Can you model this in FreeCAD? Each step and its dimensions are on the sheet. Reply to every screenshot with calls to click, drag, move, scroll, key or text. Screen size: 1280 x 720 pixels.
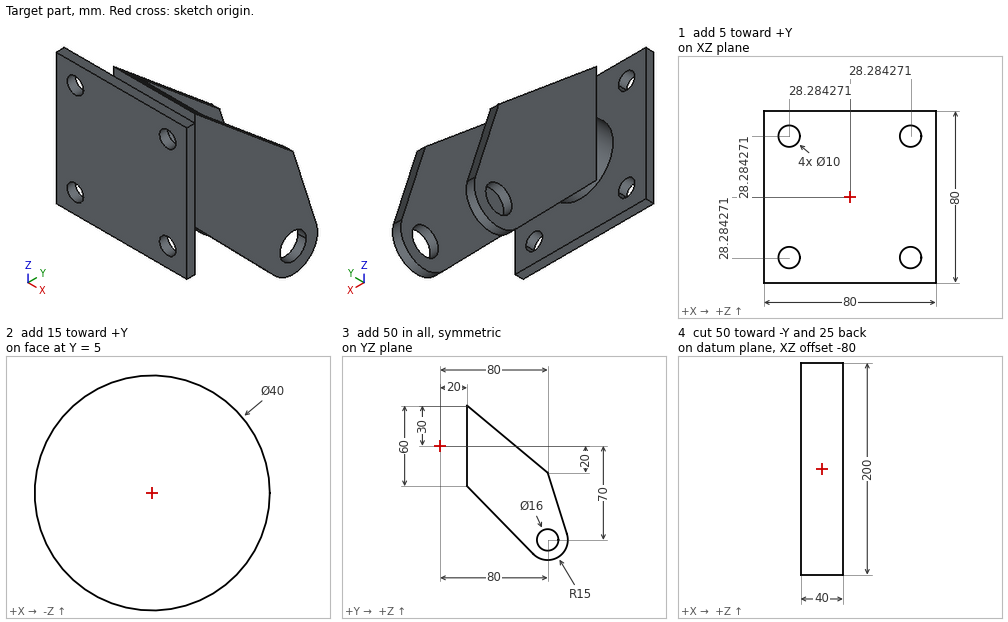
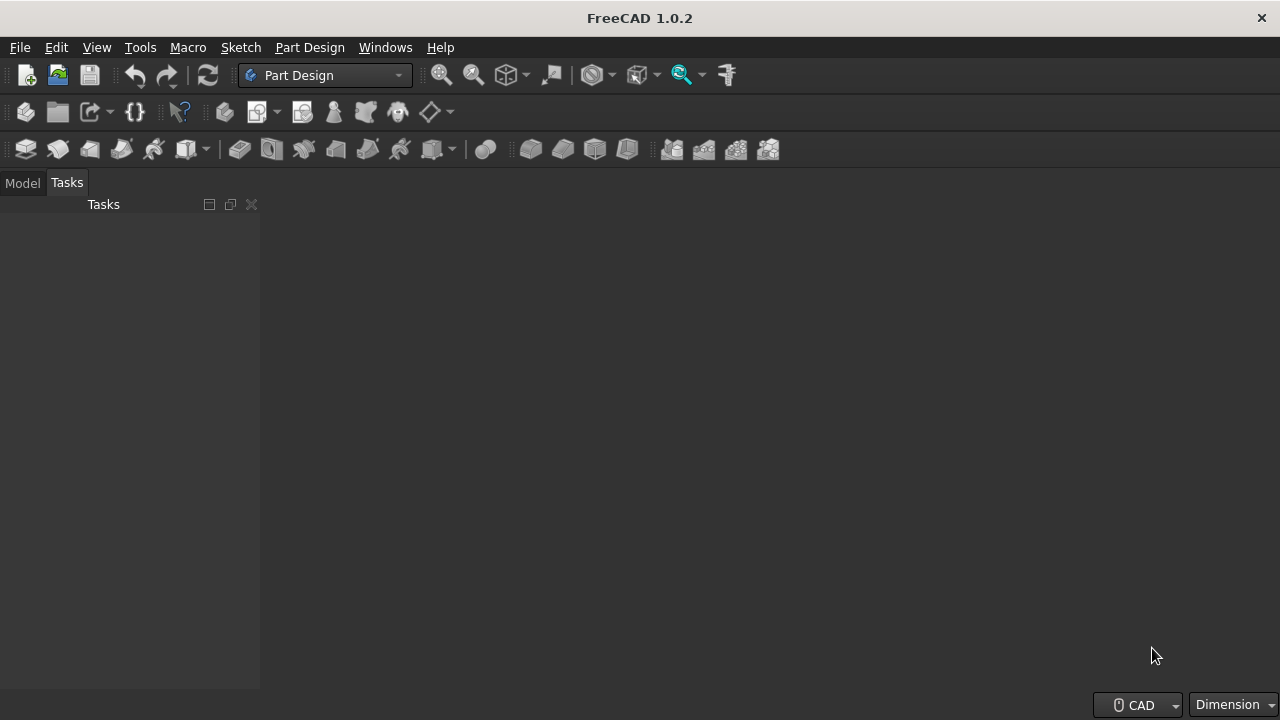
click(26, 76)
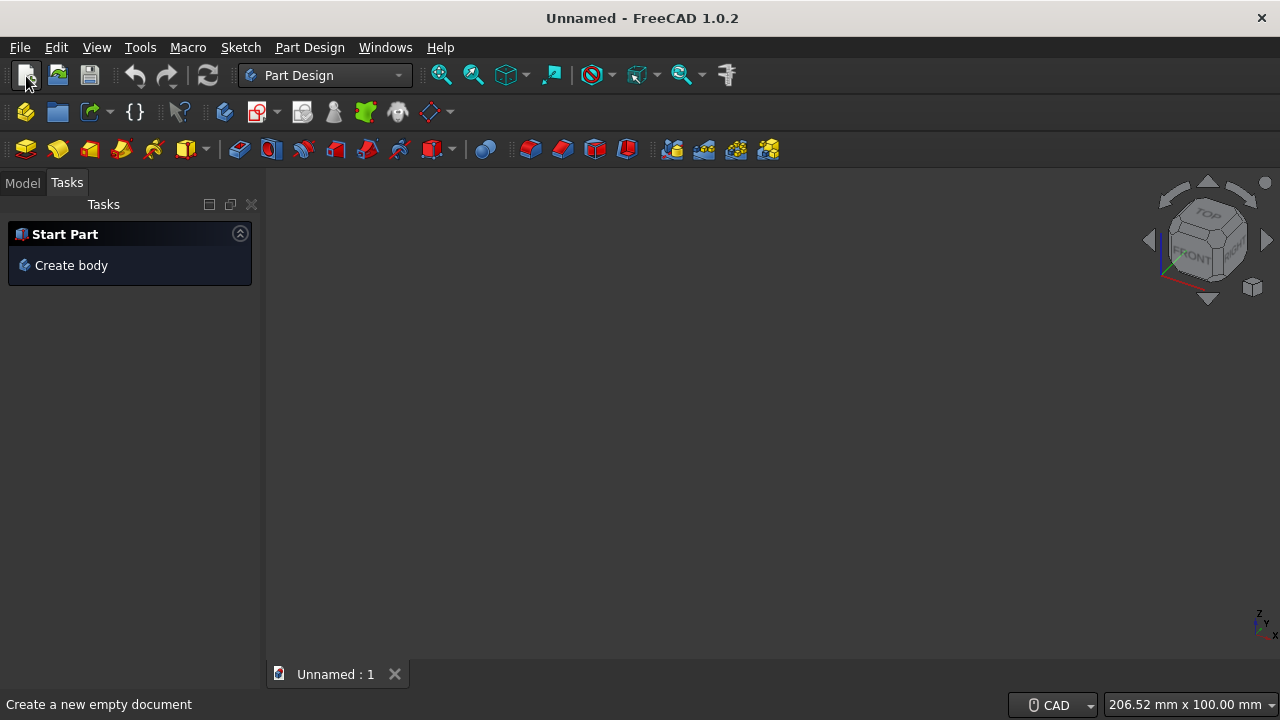
click(258, 112)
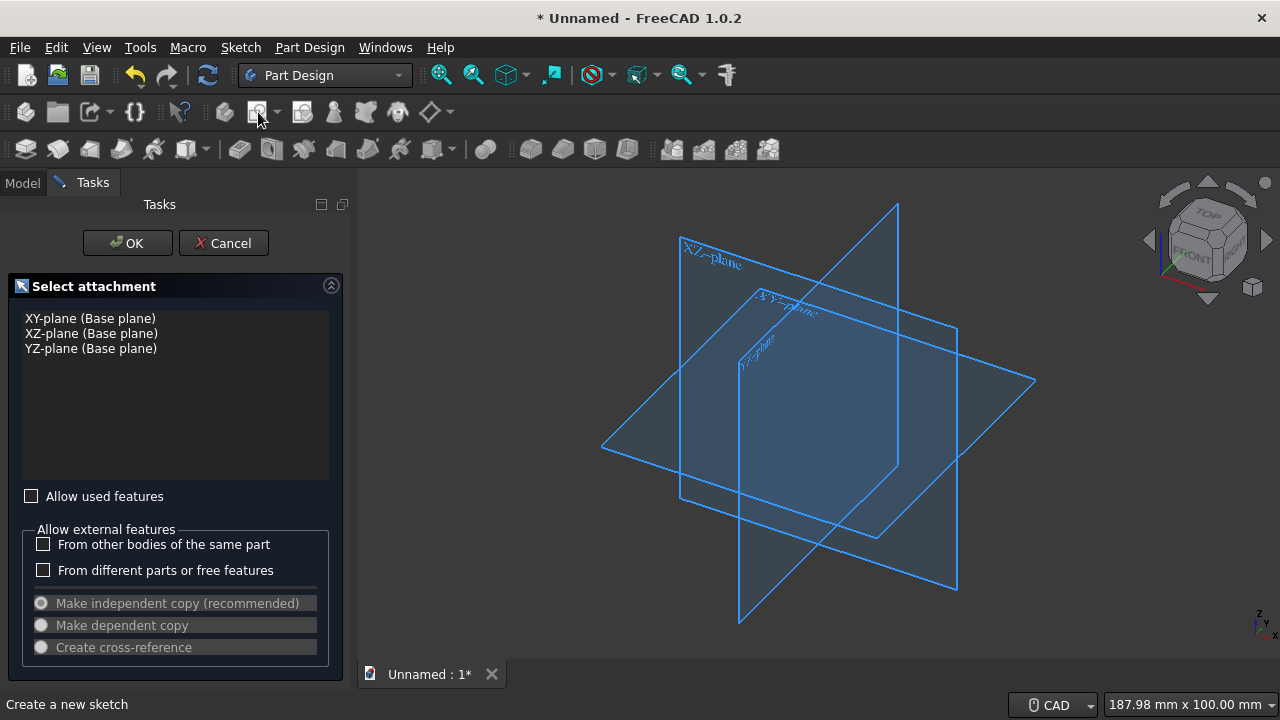
click(82, 334)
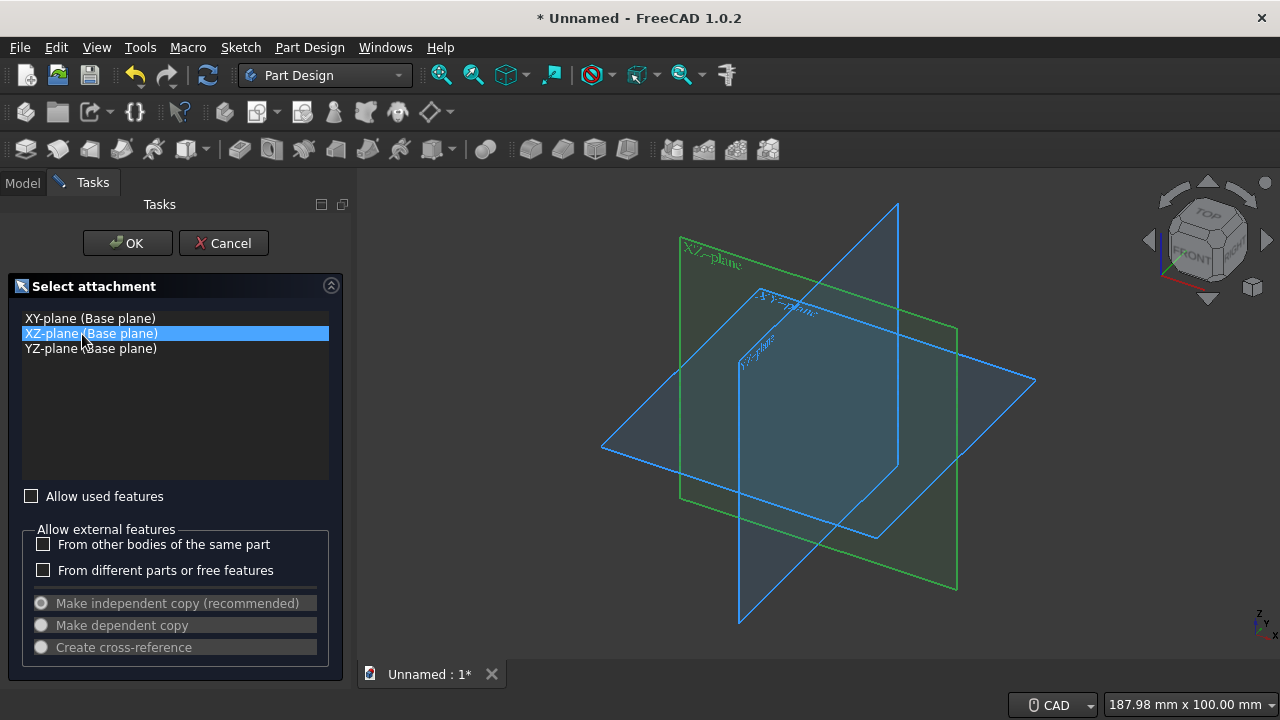
click(128, 243)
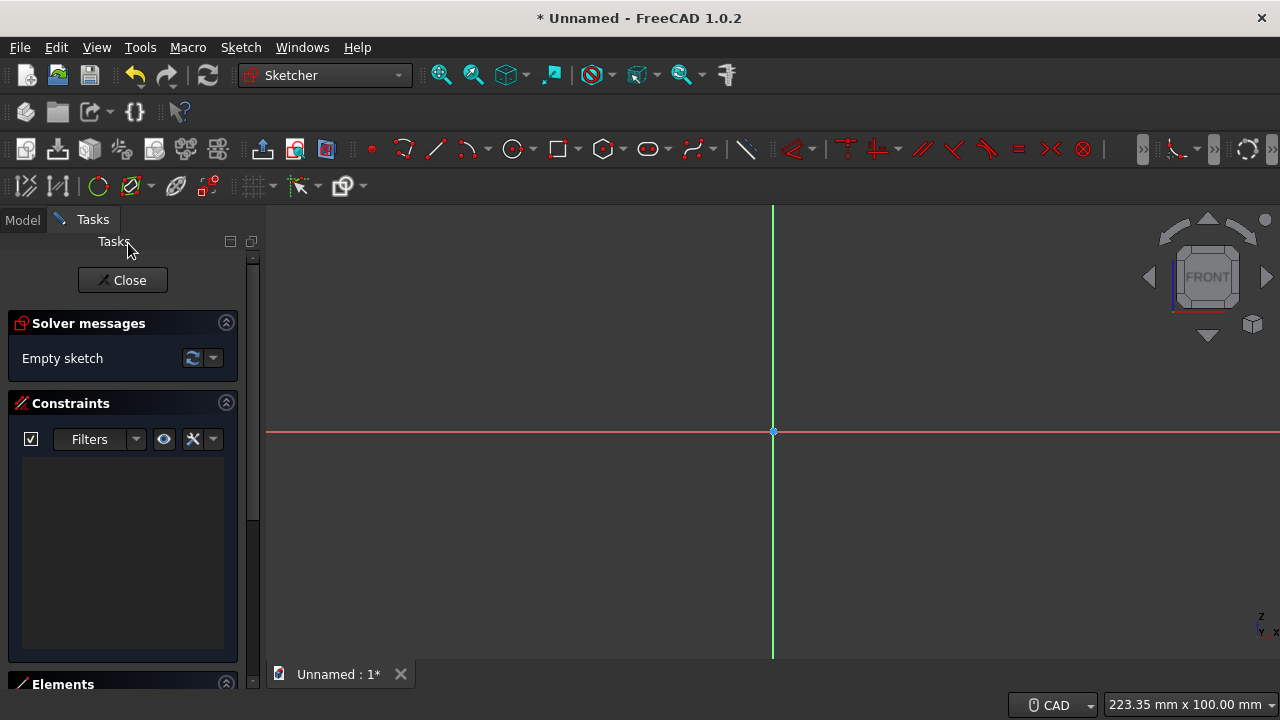
scroll(395, 432, down, 1)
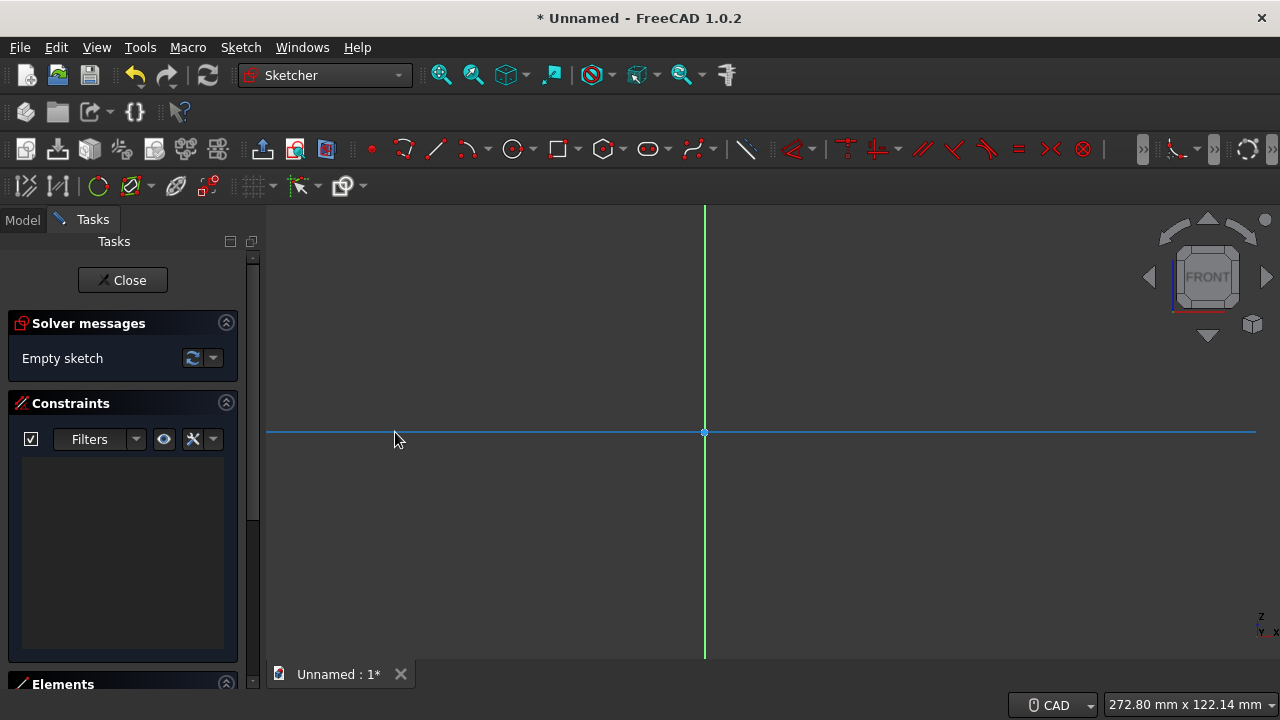
key(g)
key(v)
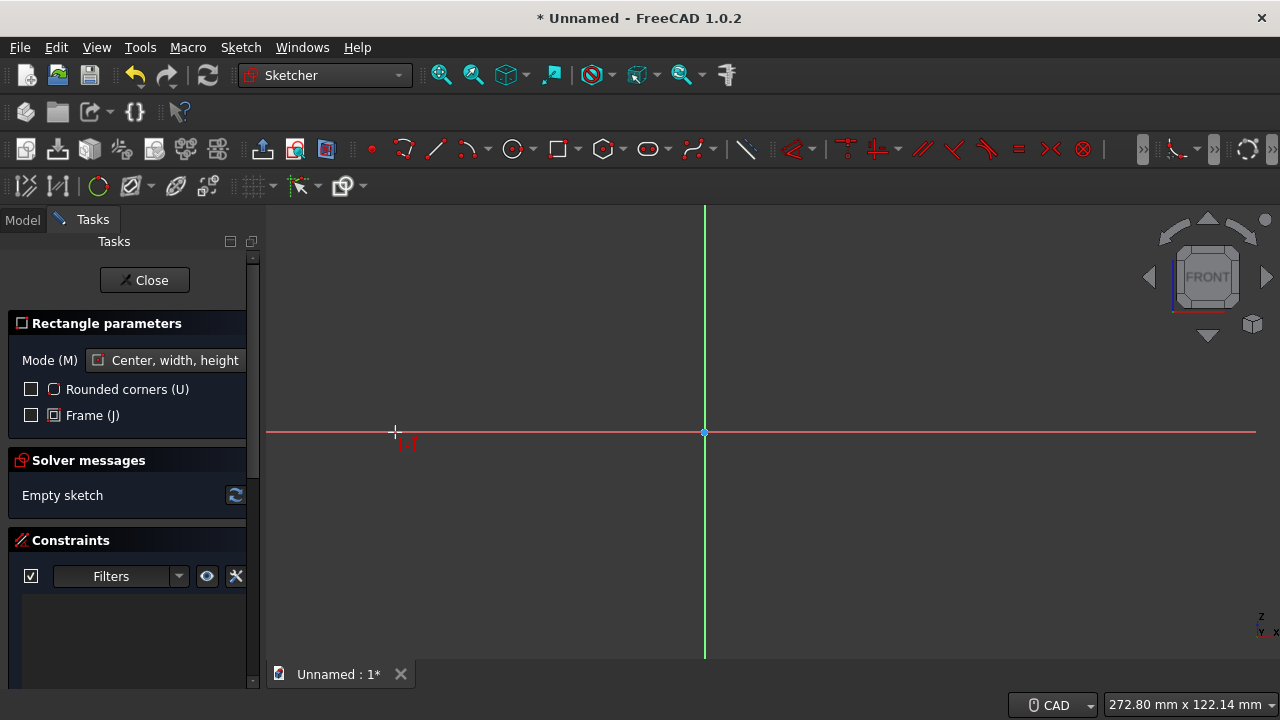
click(705, 432)
click(853, 283)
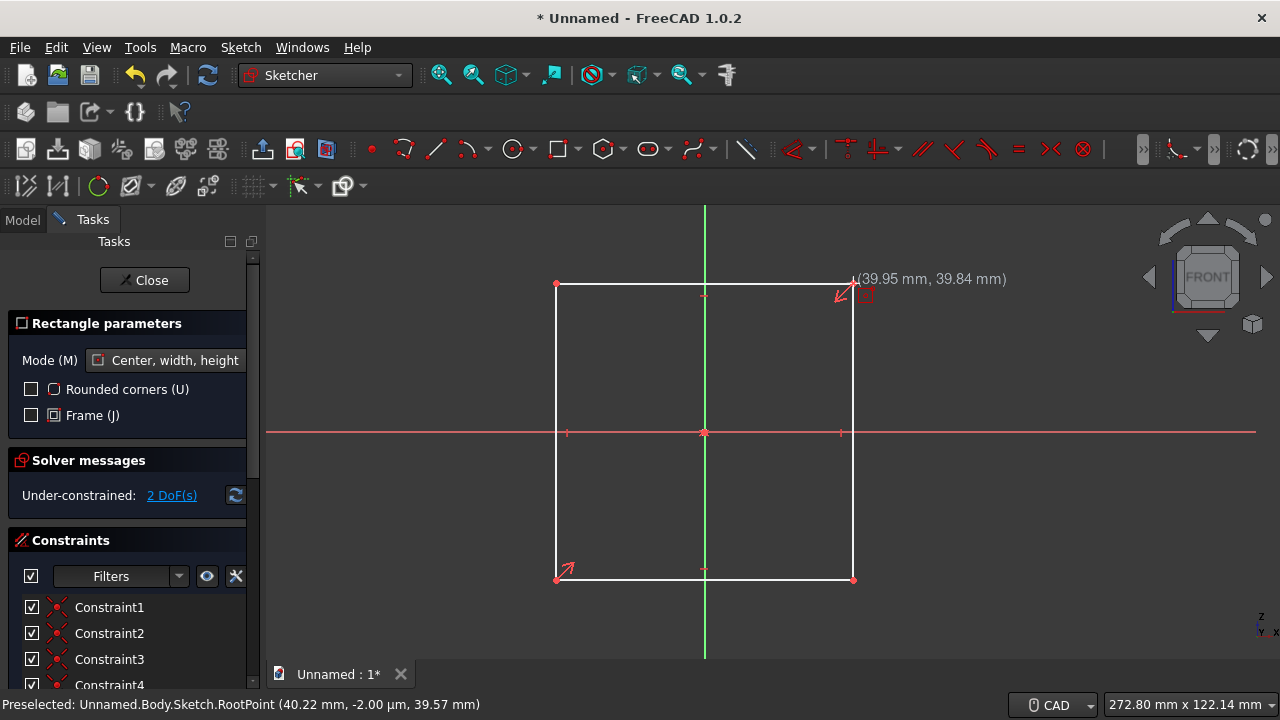
click(514, 150)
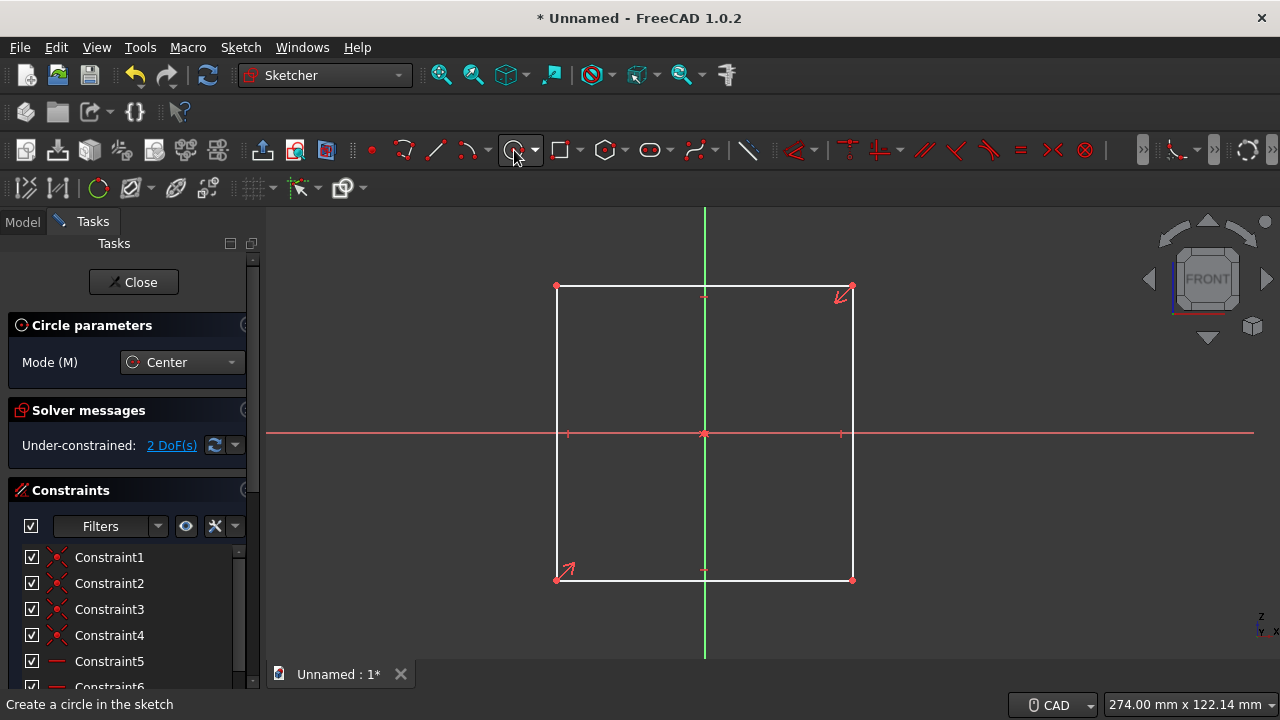
scroll(600, 328, up, 2)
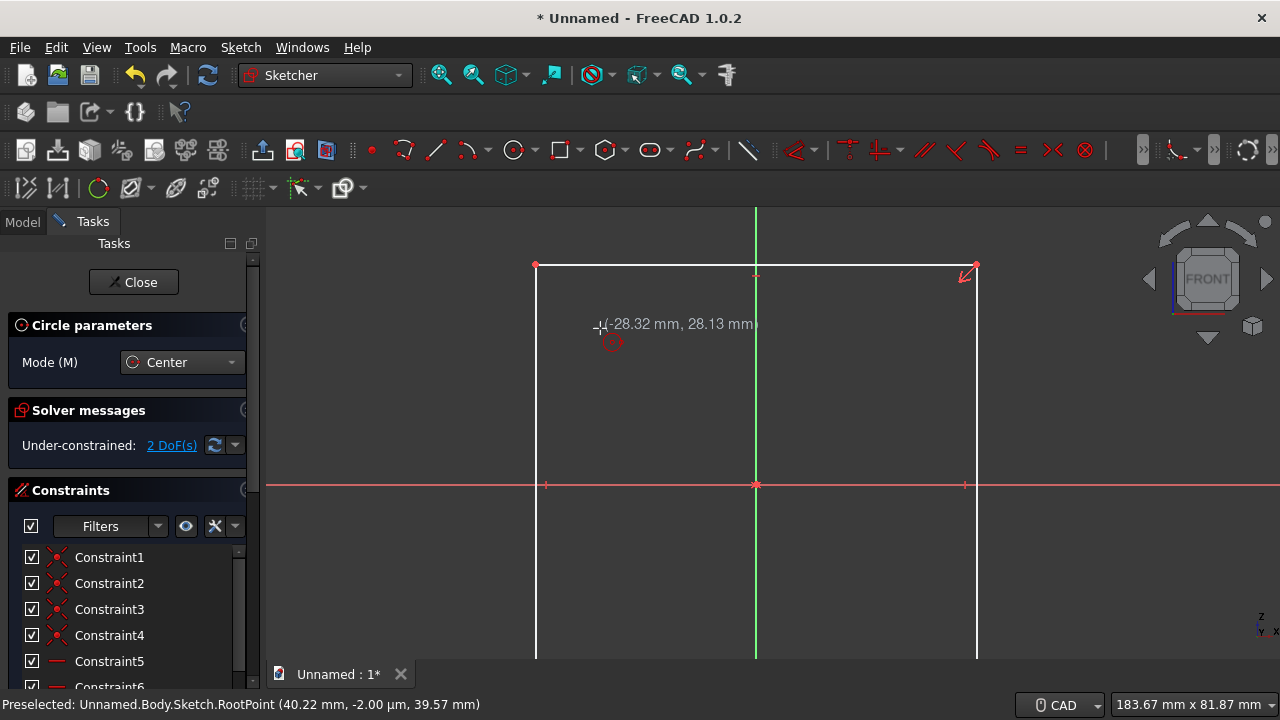
click(600, 328)
click(620, 309)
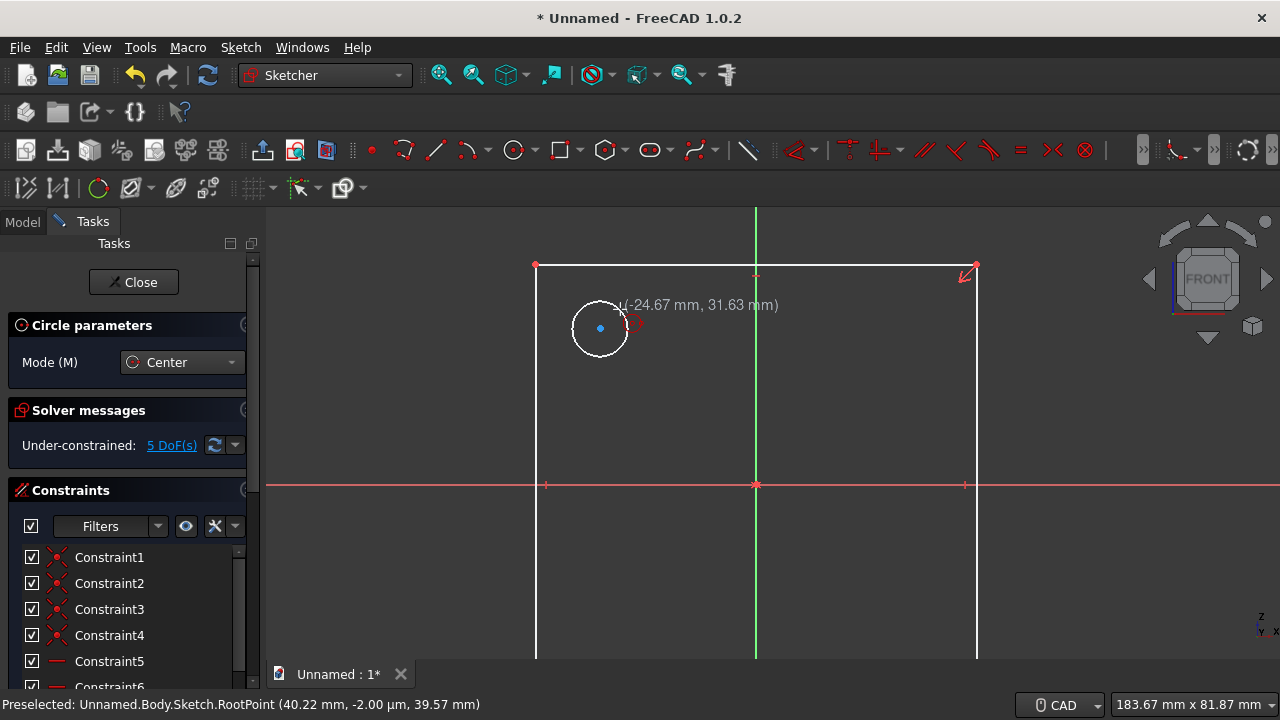
click(912, 328)
click(932, 309)